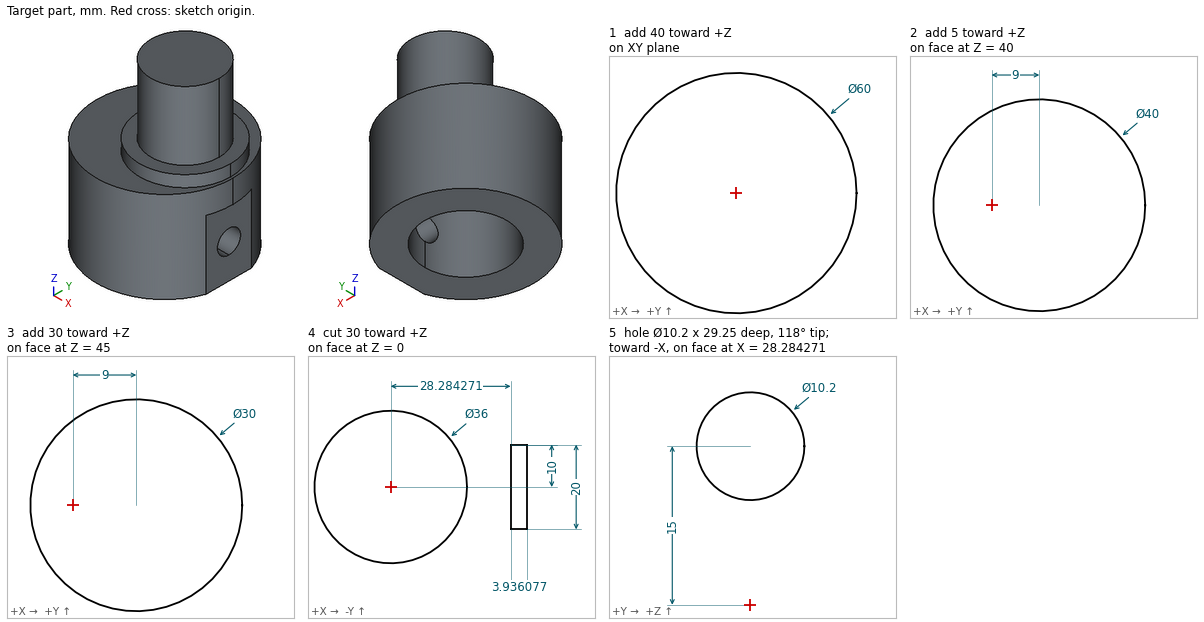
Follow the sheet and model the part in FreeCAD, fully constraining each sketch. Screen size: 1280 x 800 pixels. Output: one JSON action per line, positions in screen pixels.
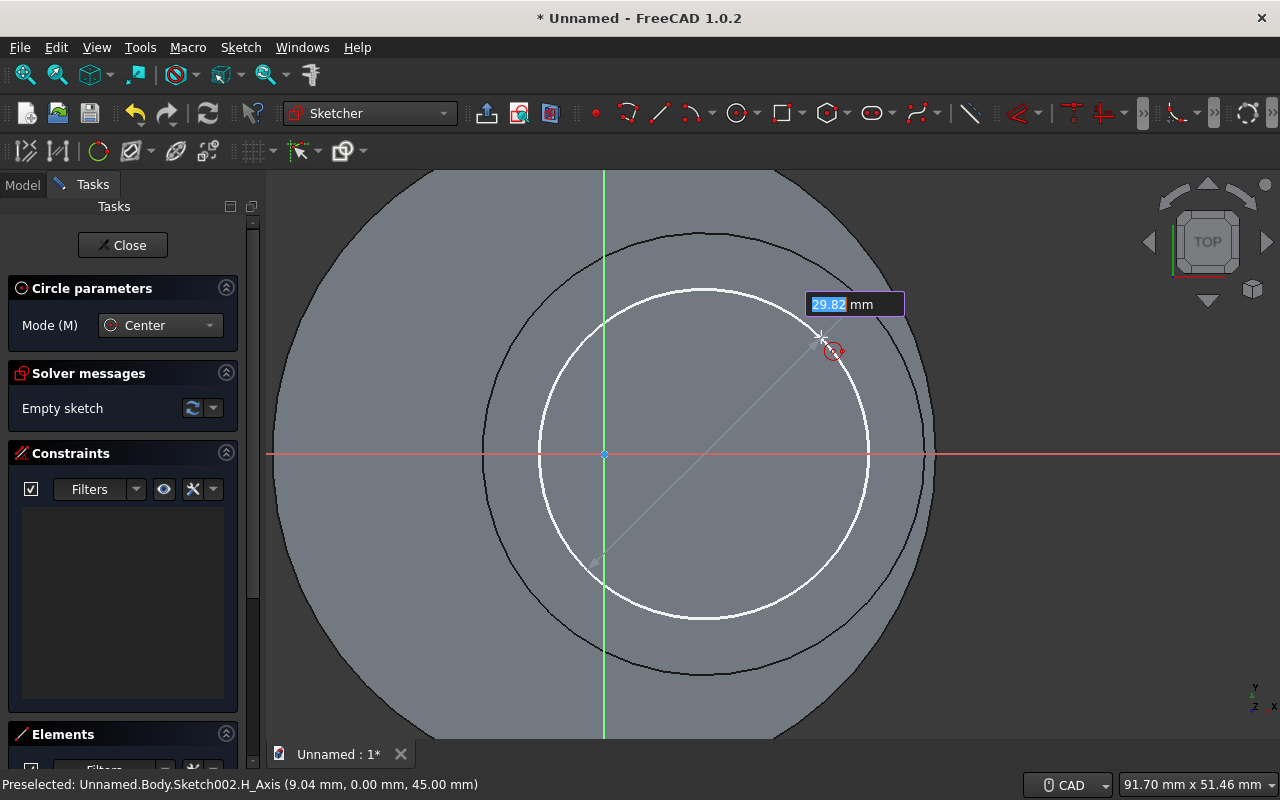
{"action": "type", "text": "30"}
{"action": "key", "text": "Return"}
{"action": "key", "text": "Escape"}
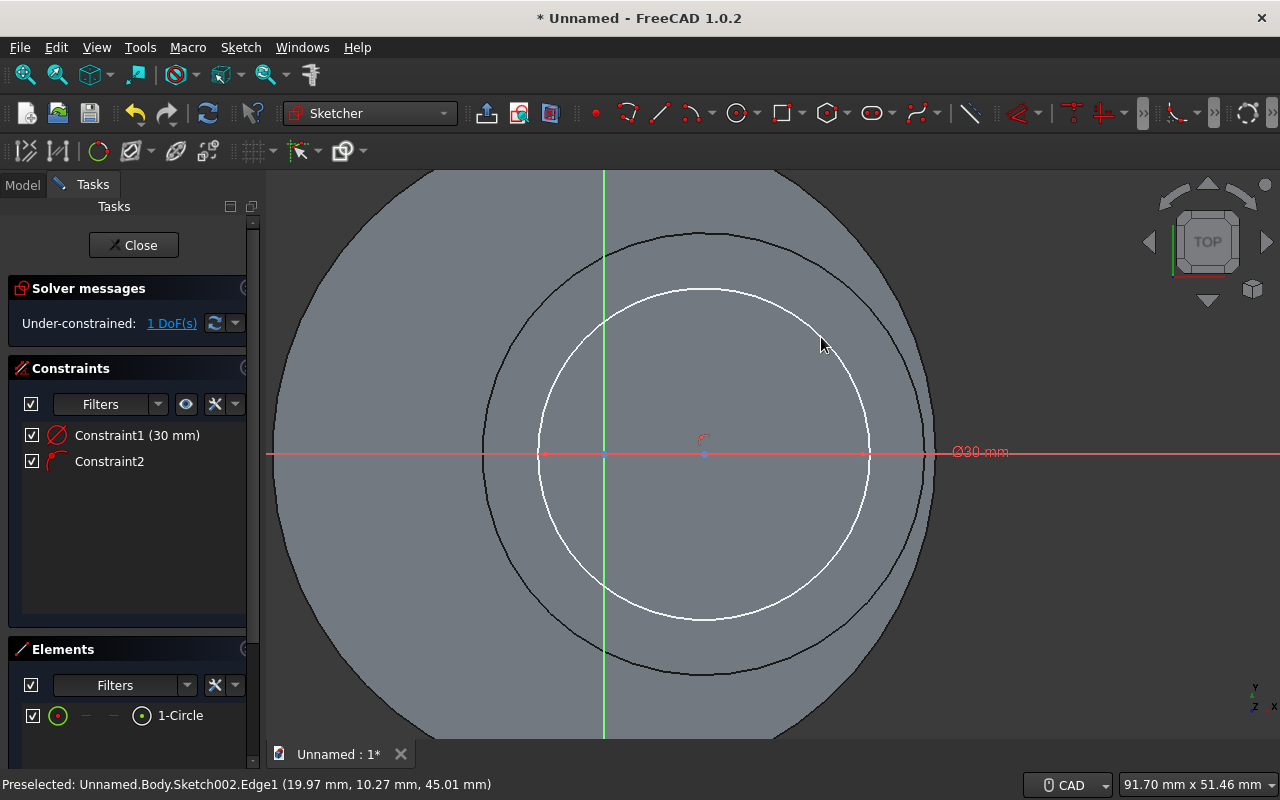
{"action": "left_click", "coordinate": [1018, 114]}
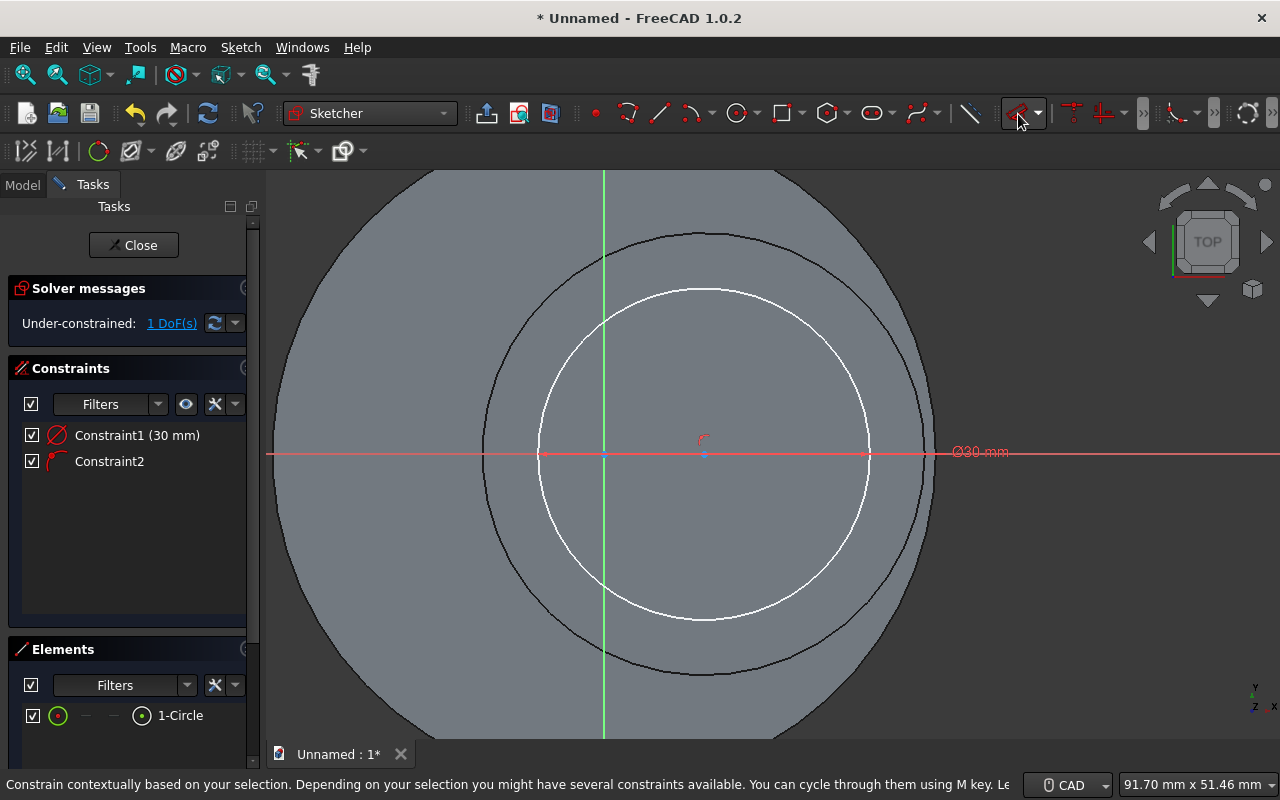
{"action": "left_click", "coordinate": [704, 454]}
{"action": "left_click", "coordinate": [654, 488]}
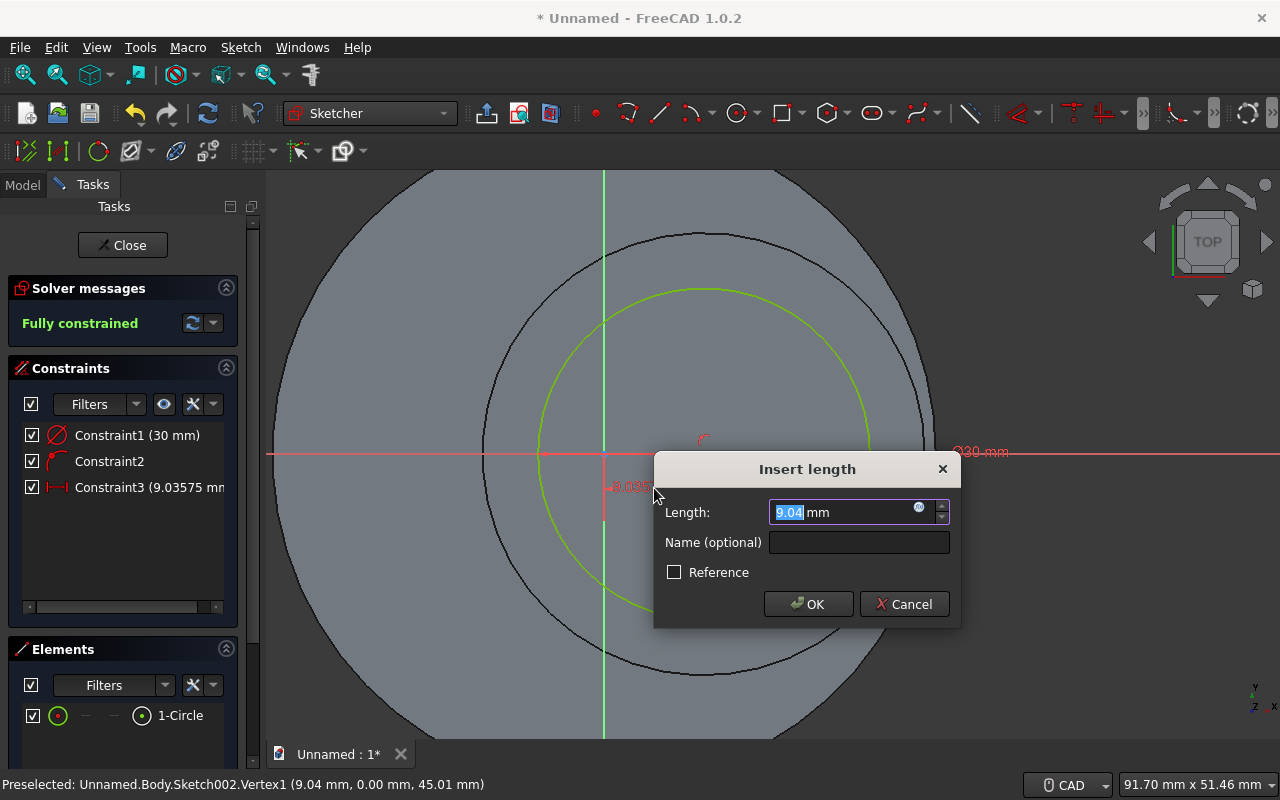
{"action": "type", "text": "9"}
{"action": "key", "text": "Return"}
{"action": "key", "text": "Escape"}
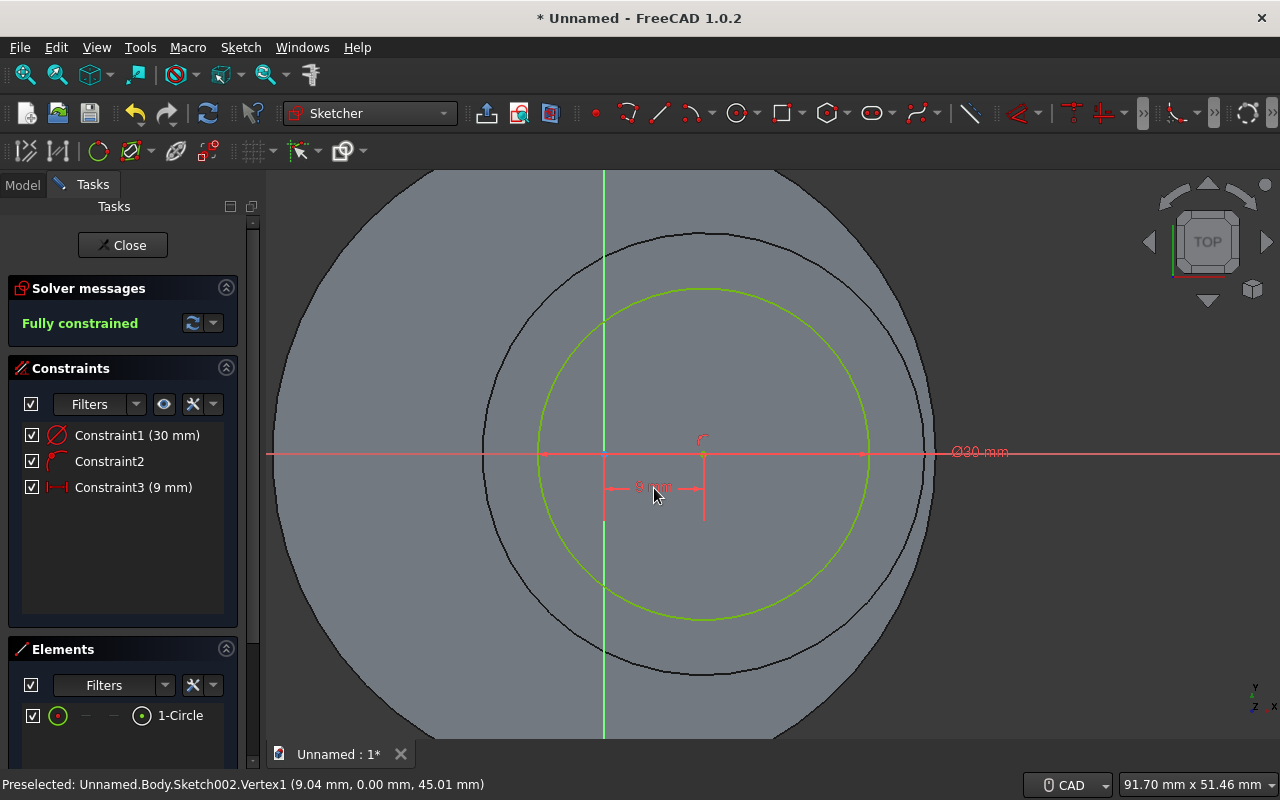
{"action": "left_click", "coordinate": [123, 245]}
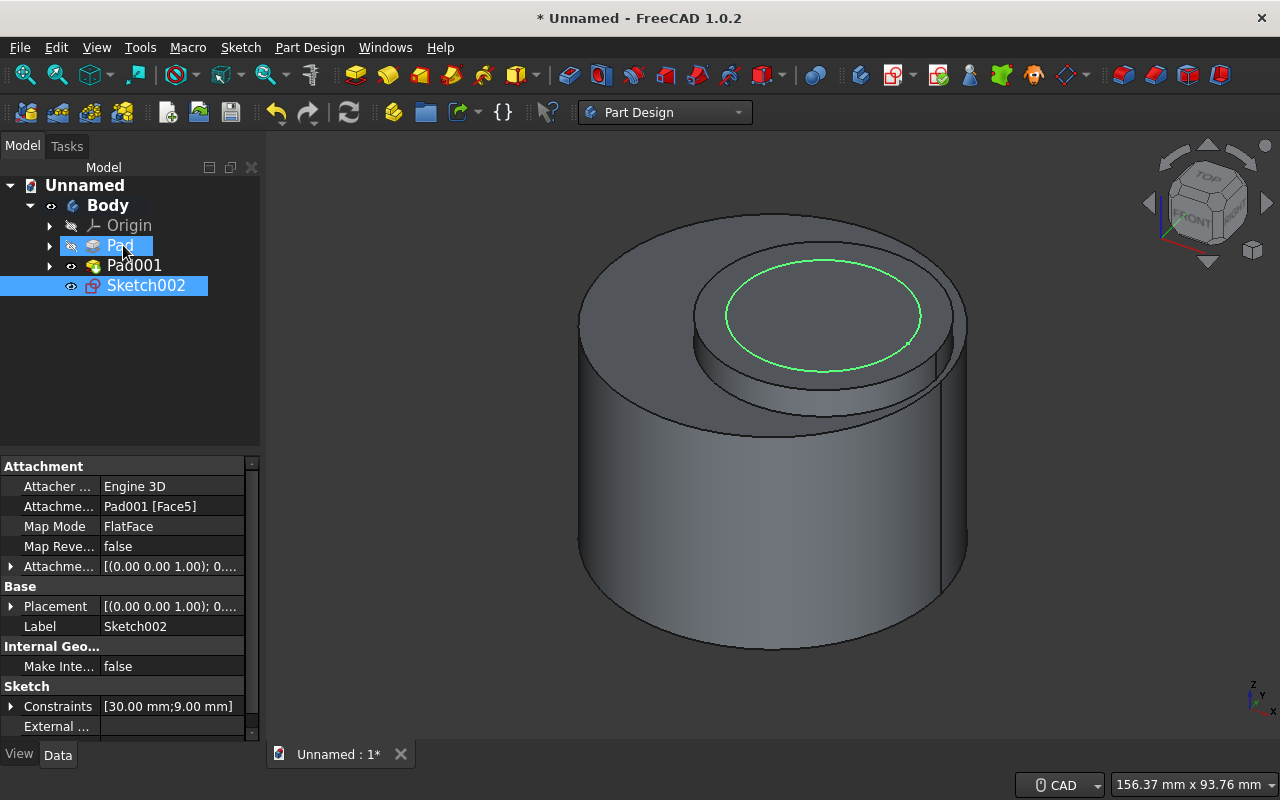
{"action": "left_click", "coordinate": [356, 76]}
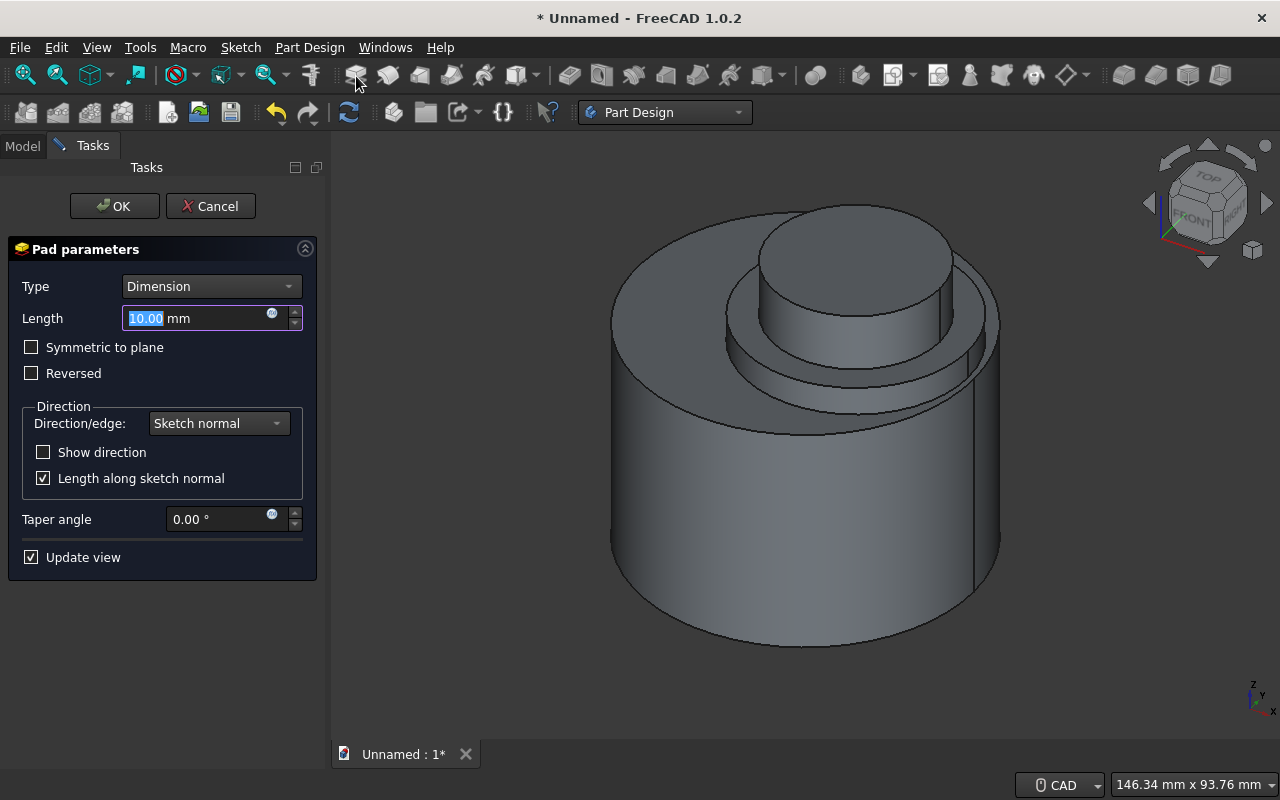
{"action": "type", "text": "30"}
{"action": "key", "text": "Tab"}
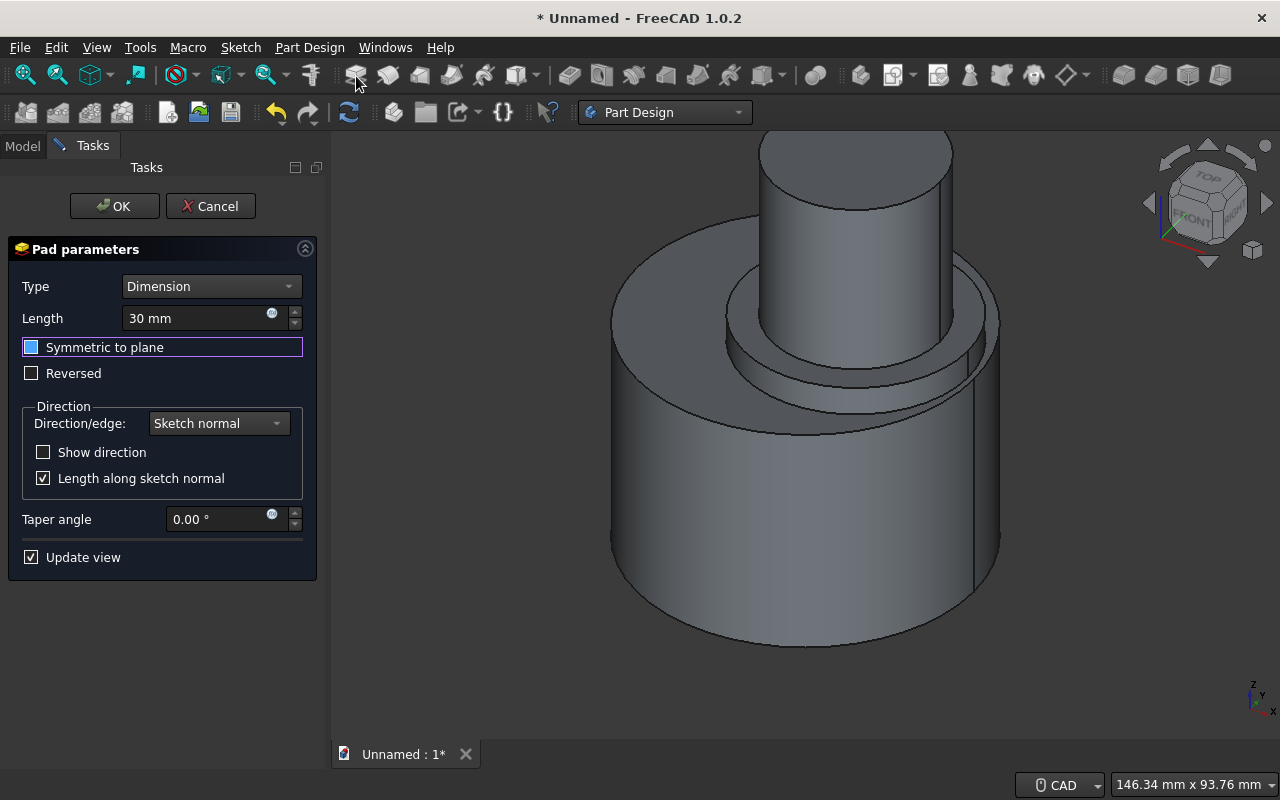
{"action": "left_click", "coordinate": [115, 206]}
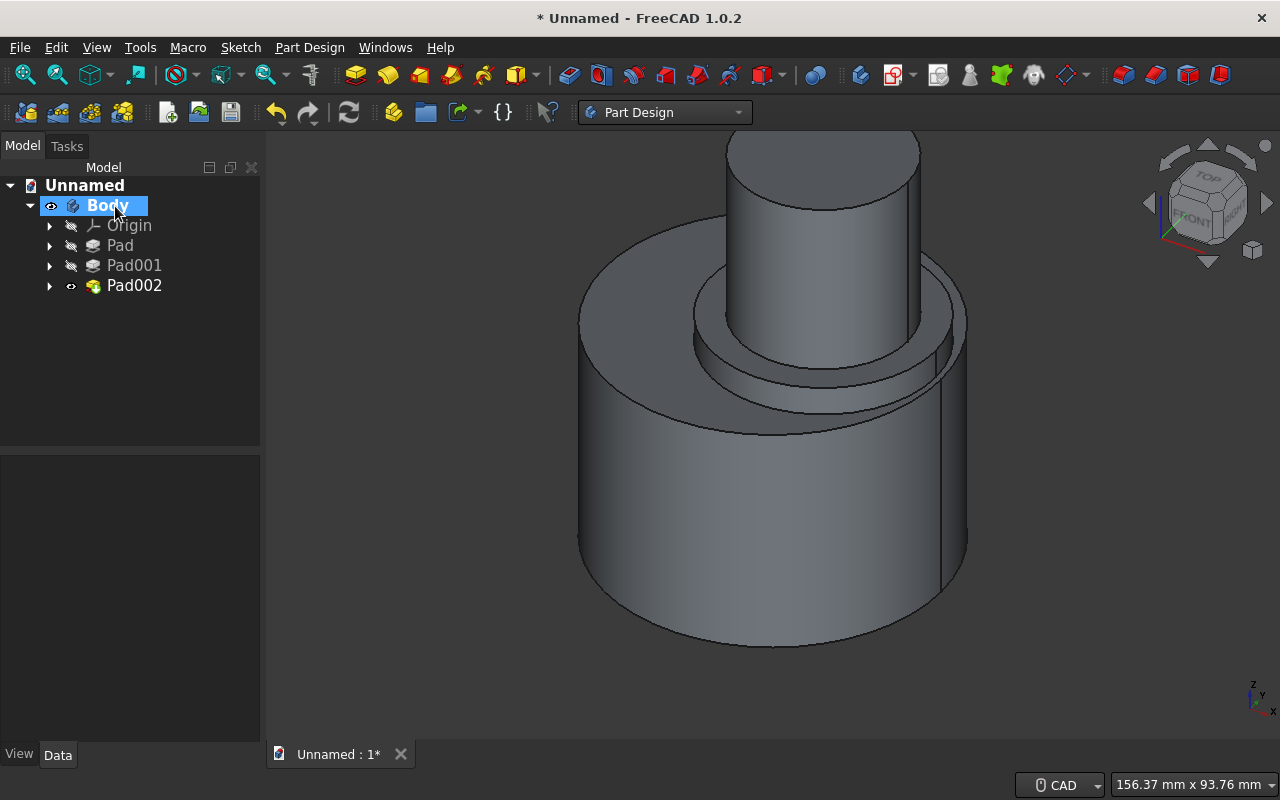
{"action": "left_click", "coordinate": [26, 76]}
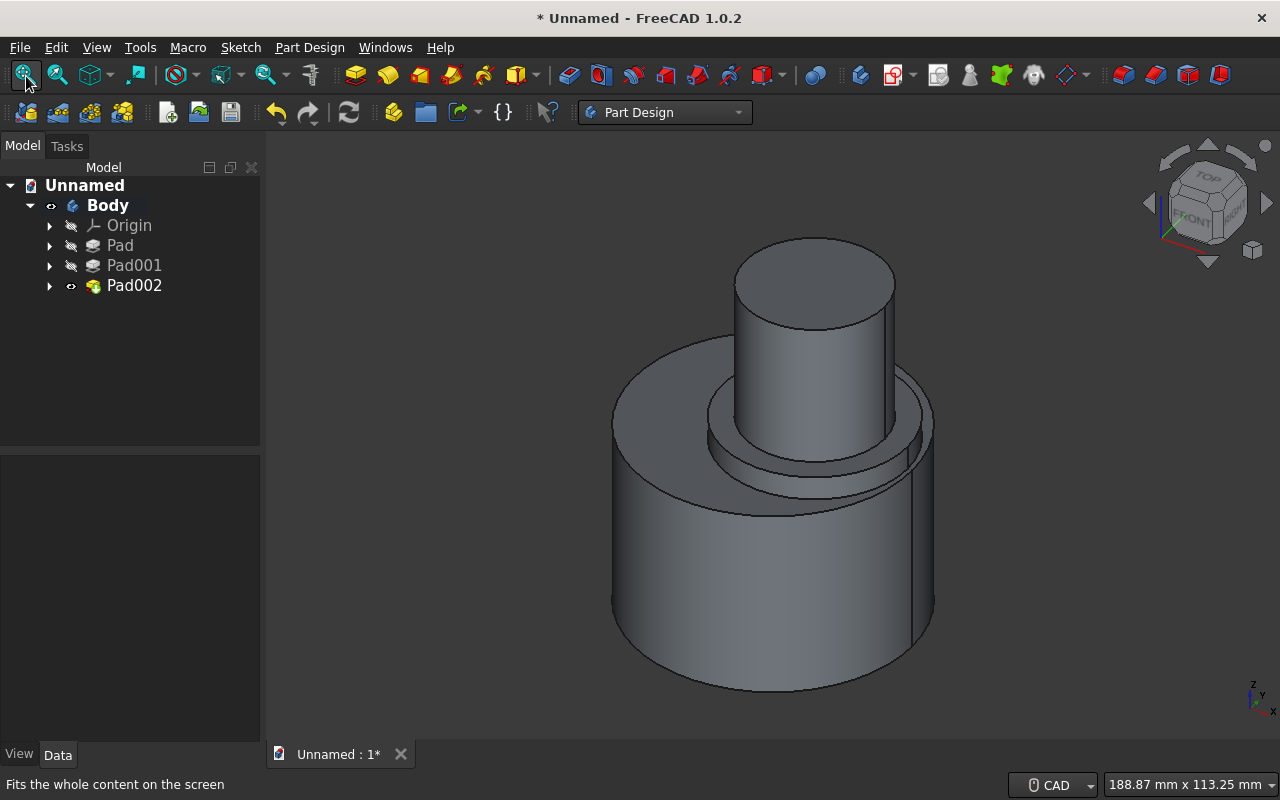
{"action": "key", "text": "5"}